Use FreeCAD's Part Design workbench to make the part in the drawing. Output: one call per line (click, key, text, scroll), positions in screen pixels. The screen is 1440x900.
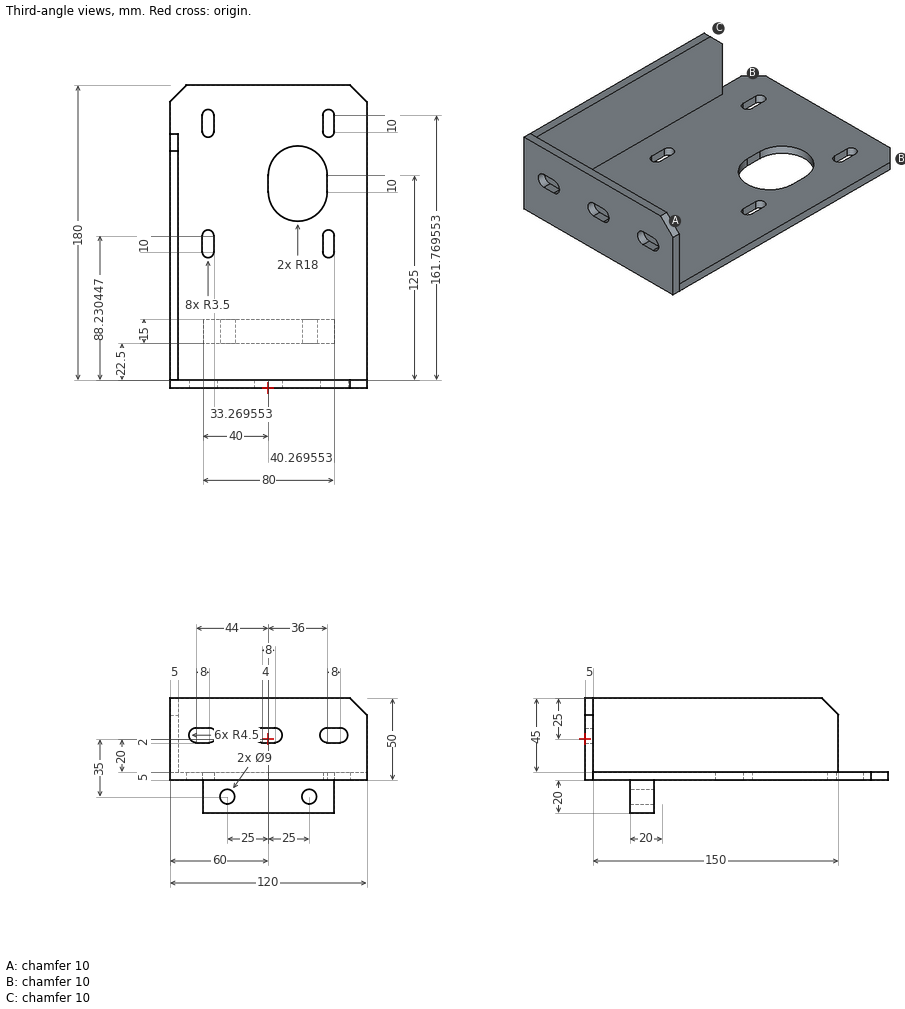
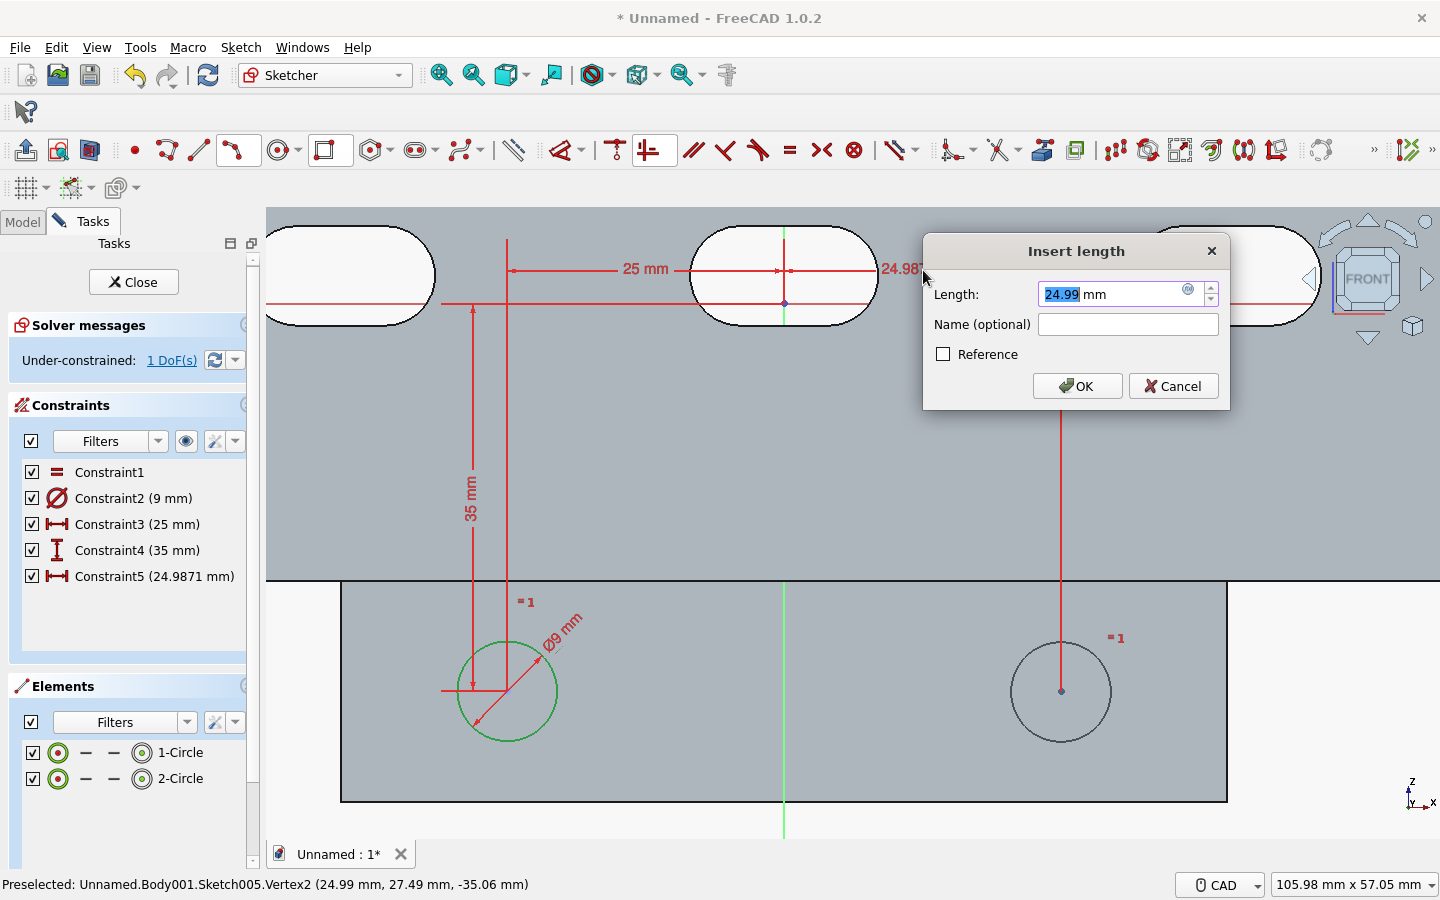
text(25)
key(Return)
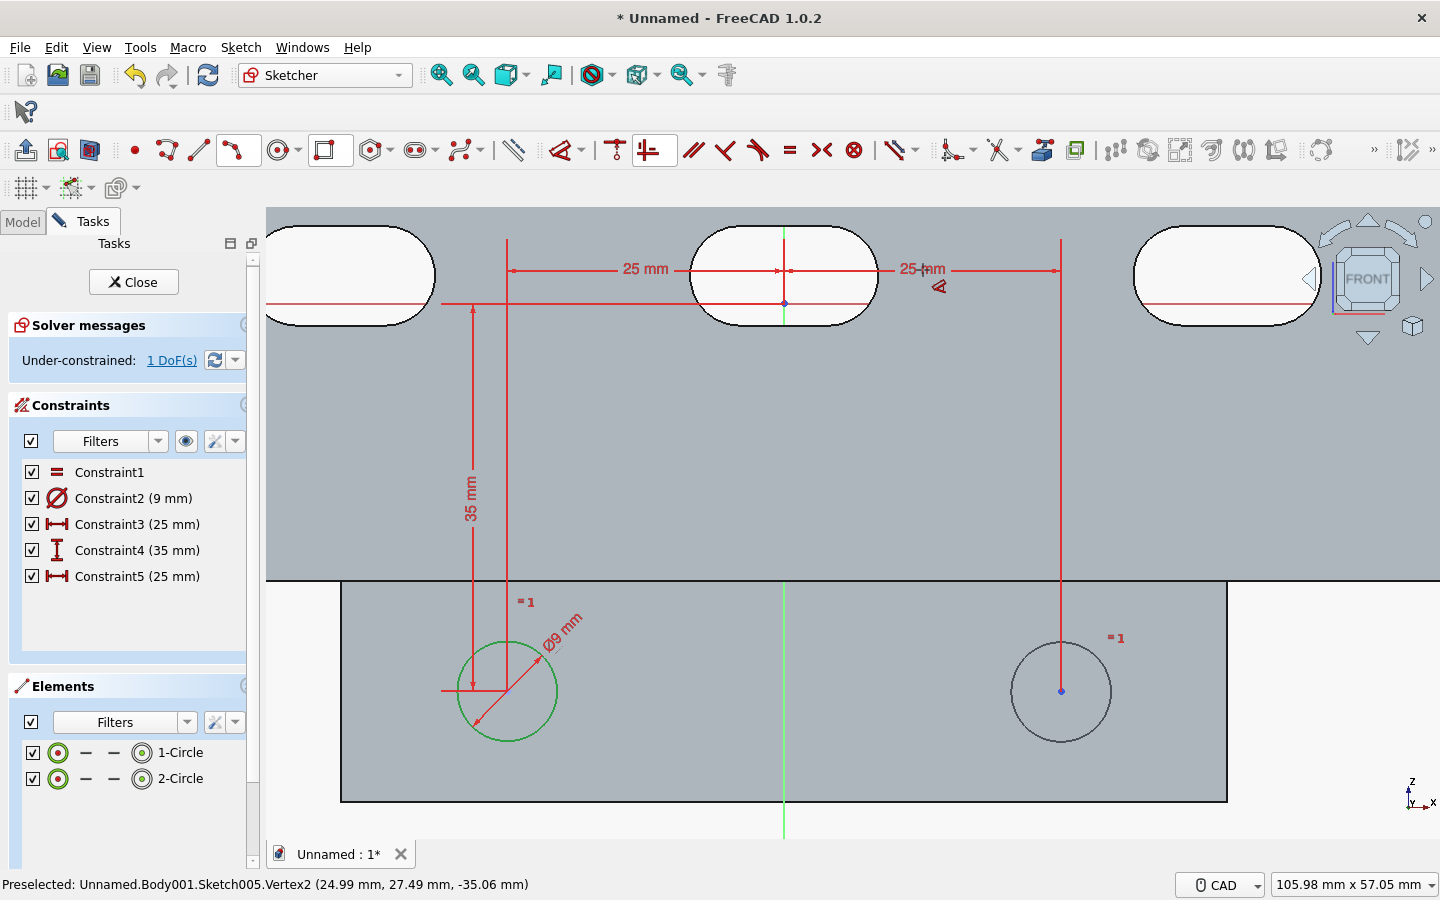
click(1061, 692)
click(1095, 498)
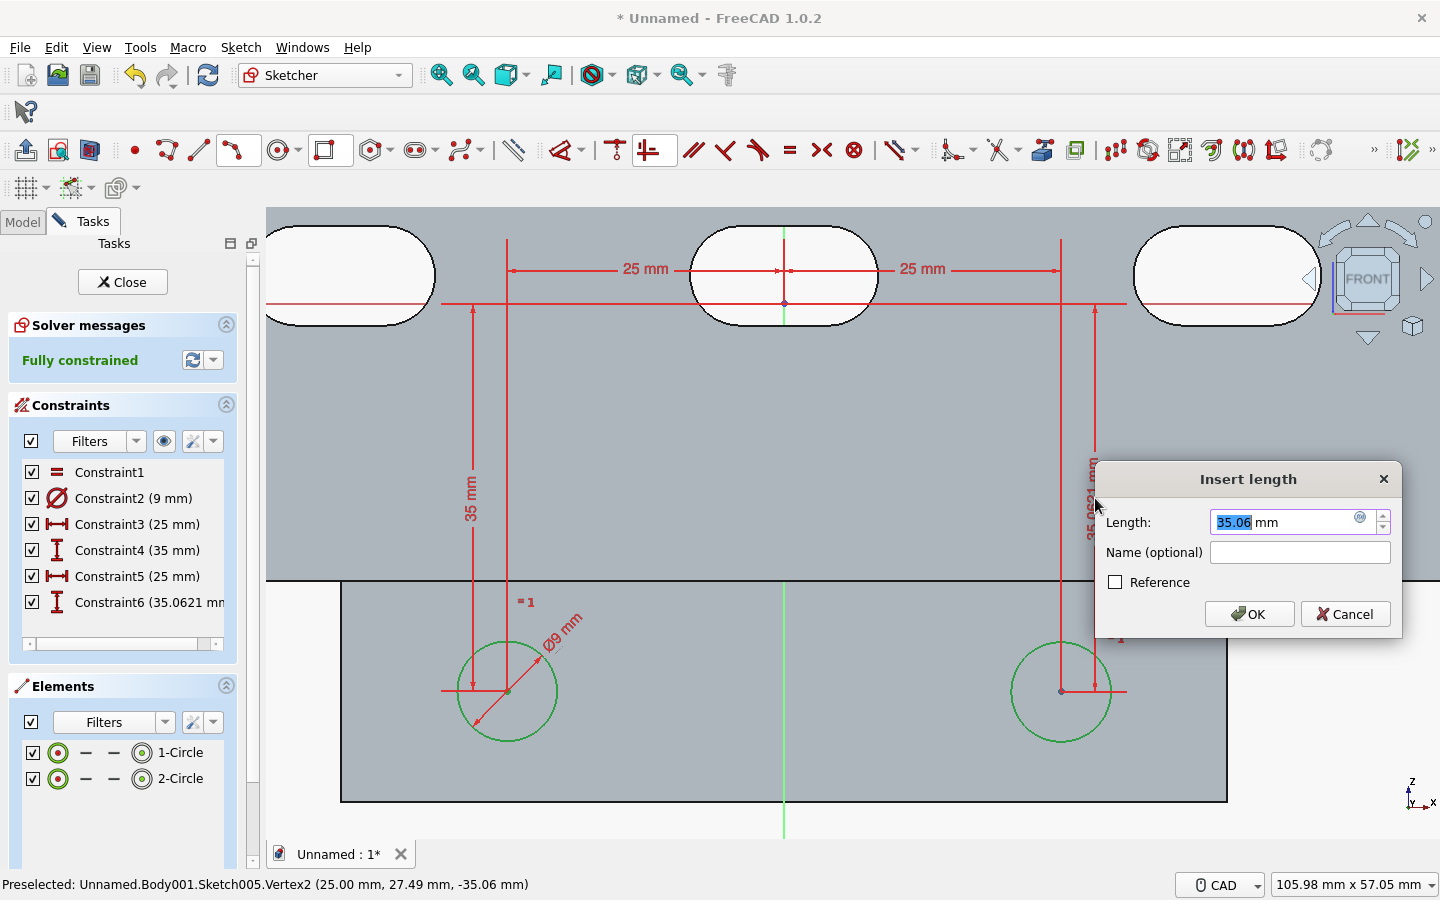
text(35)
key(Return)
key(Escape)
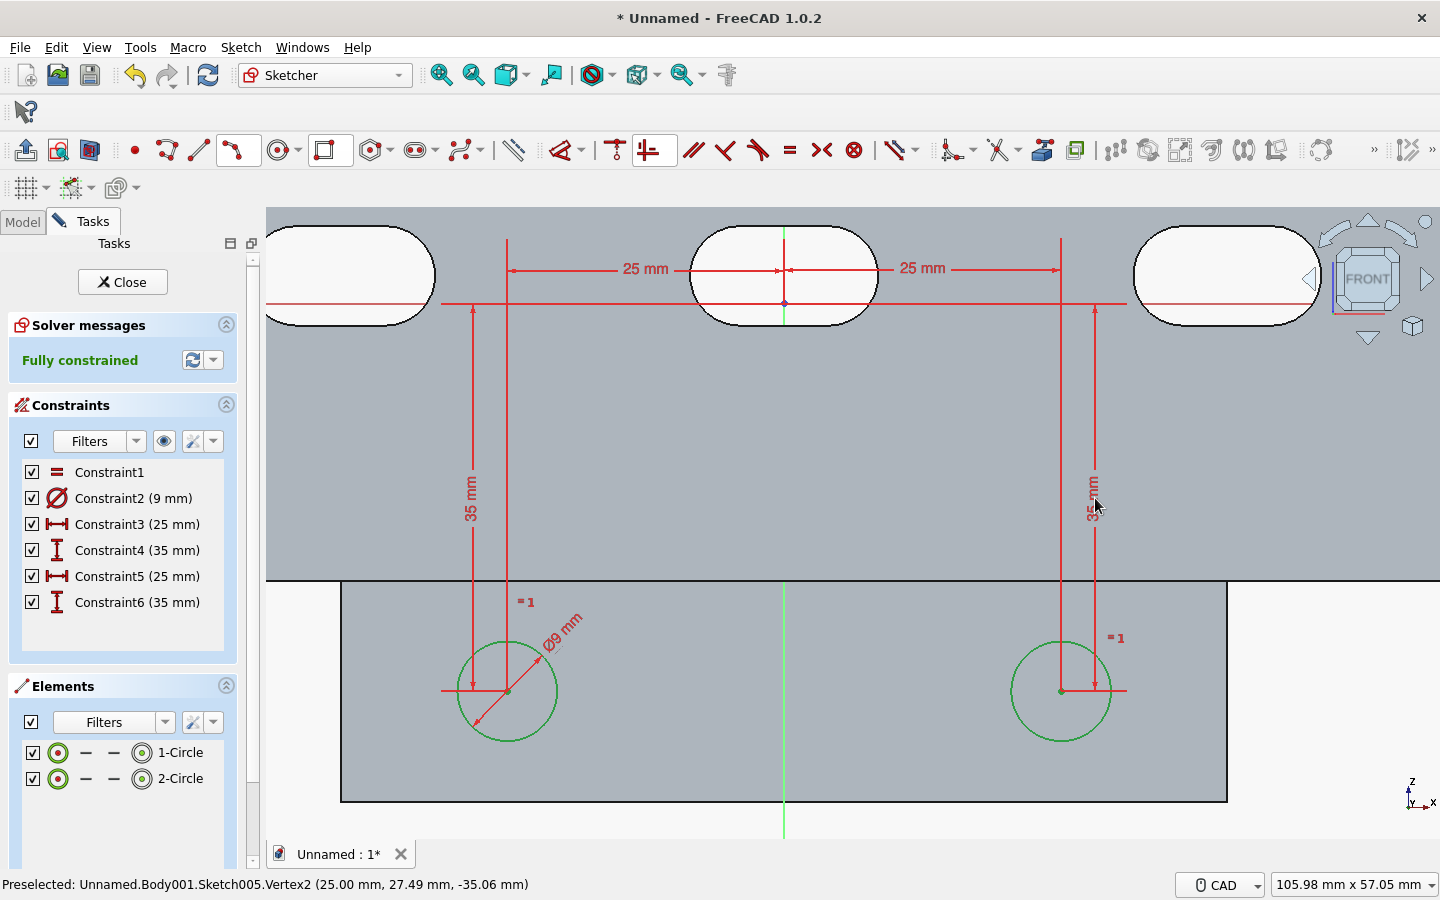
click(123, 282)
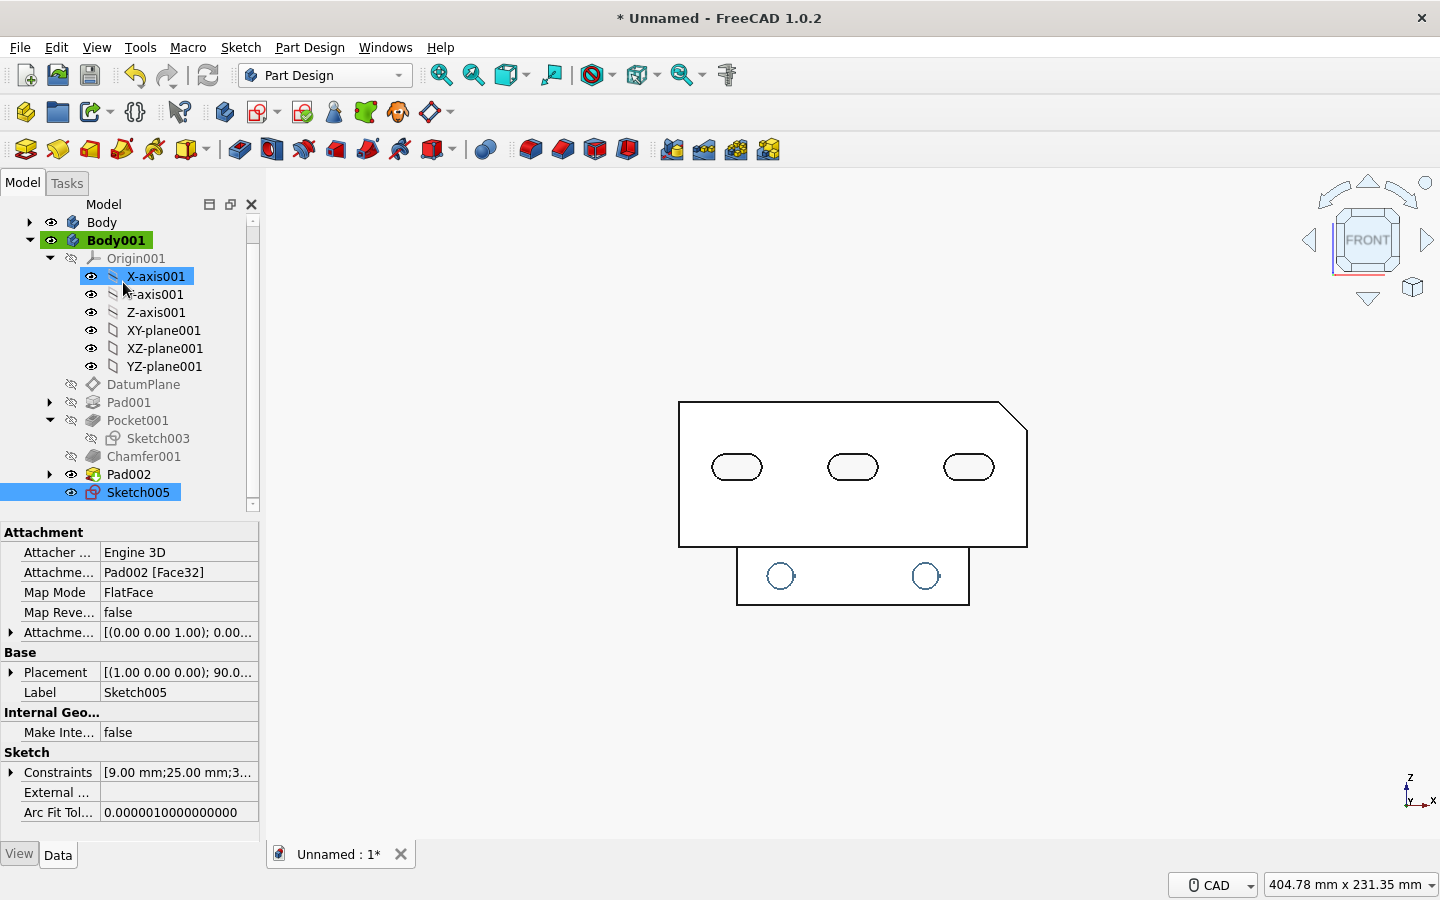
click(240, 150)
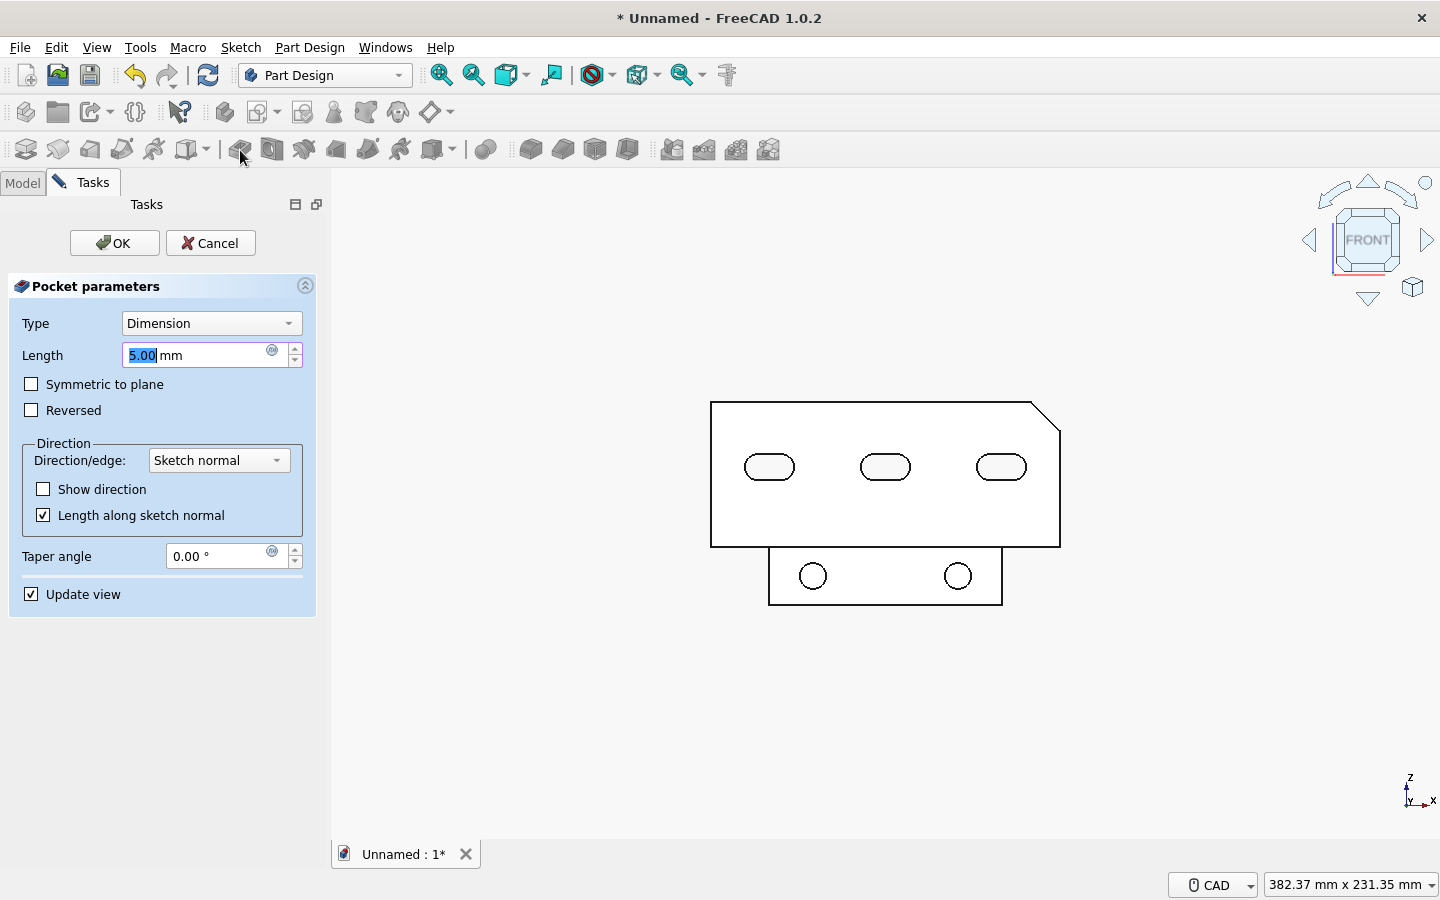
text(20)
key(Tab)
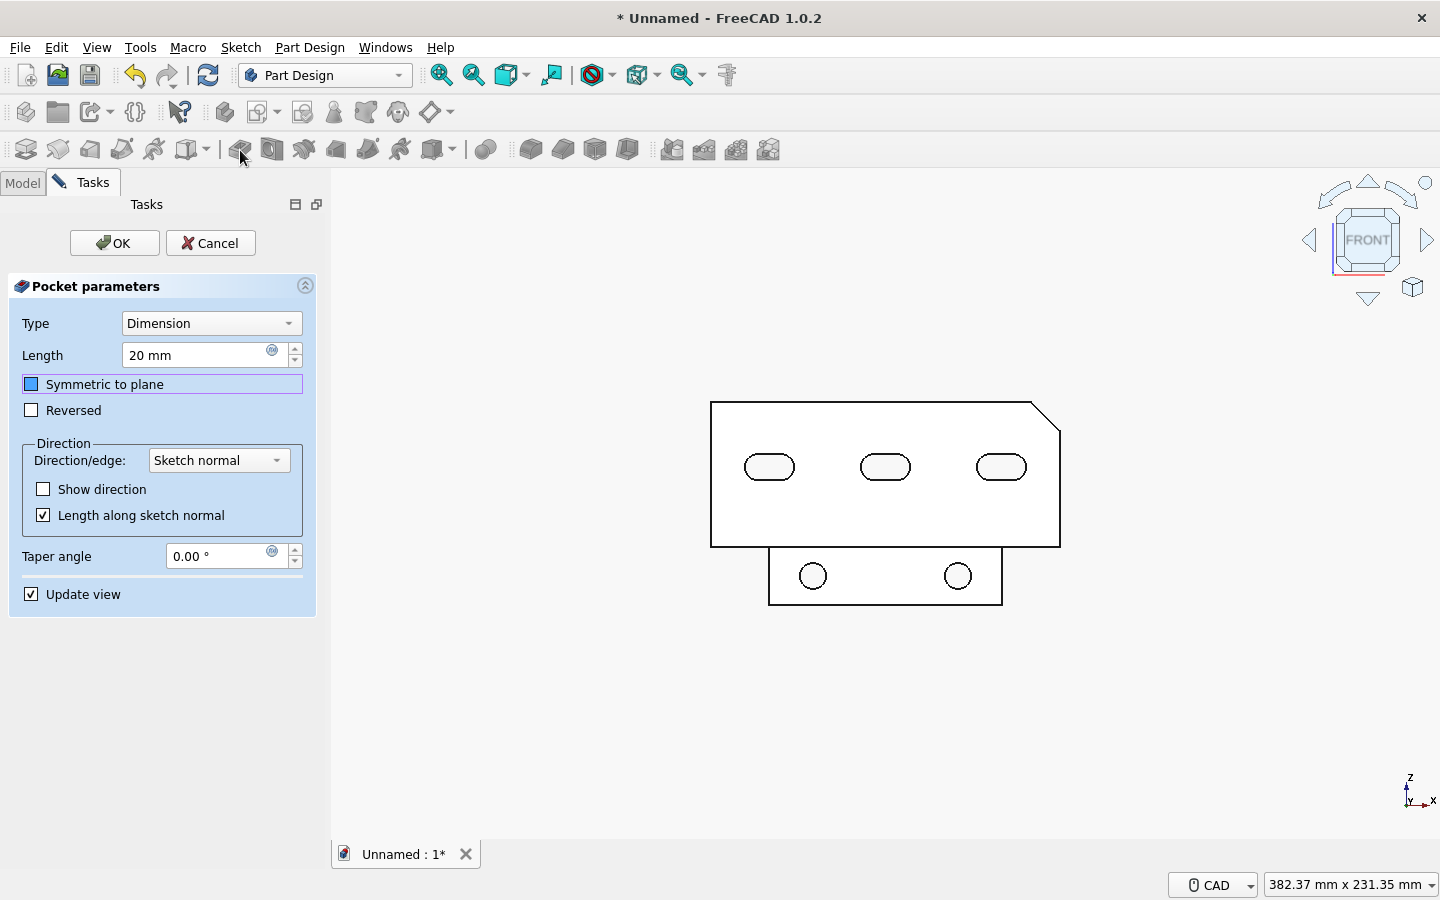
click(115, 243)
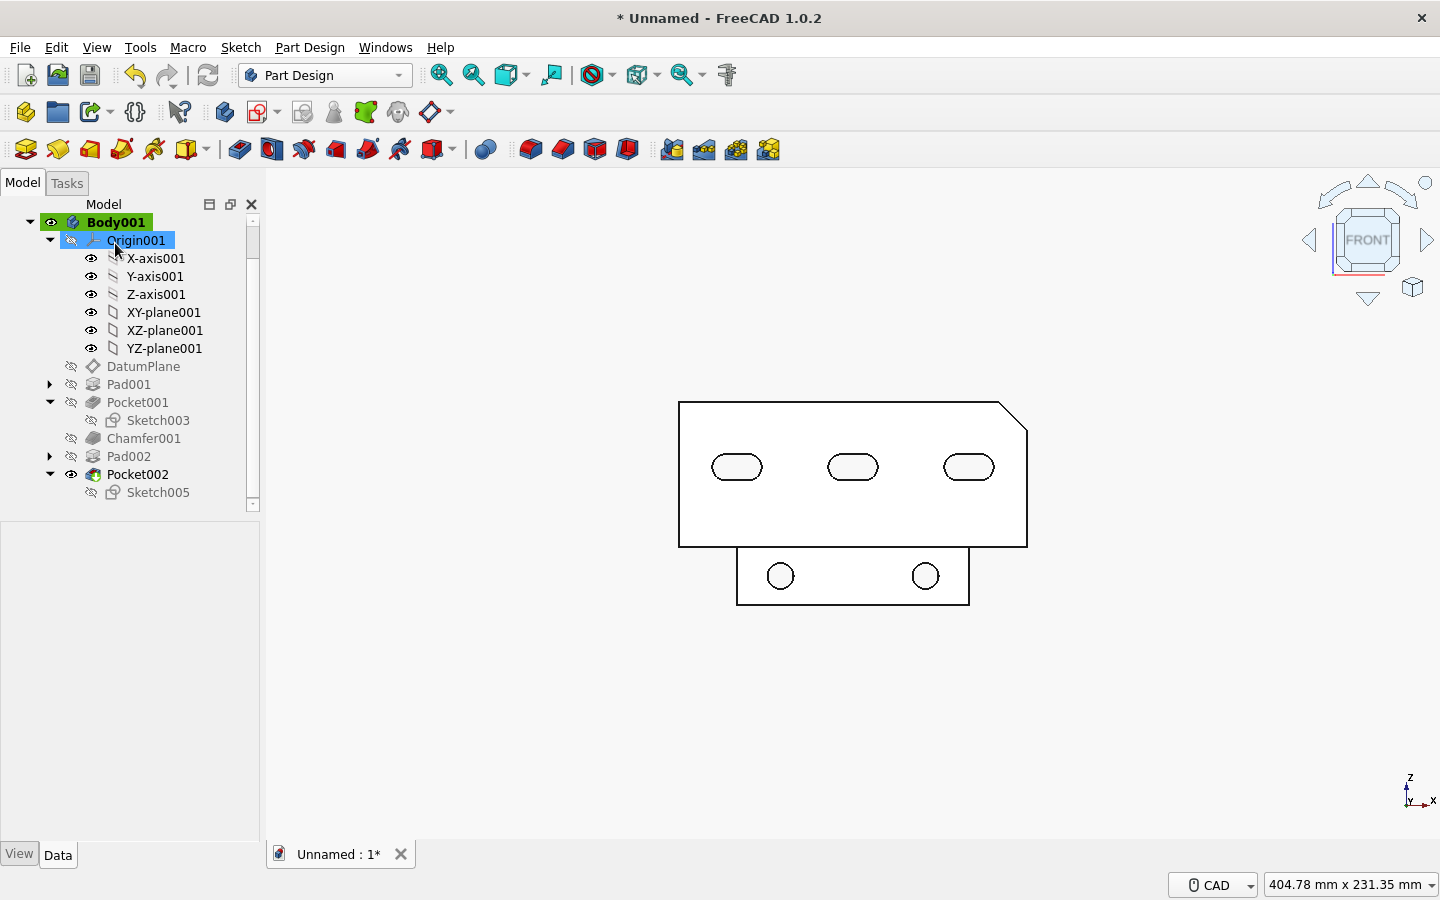
key(v)
key(f)